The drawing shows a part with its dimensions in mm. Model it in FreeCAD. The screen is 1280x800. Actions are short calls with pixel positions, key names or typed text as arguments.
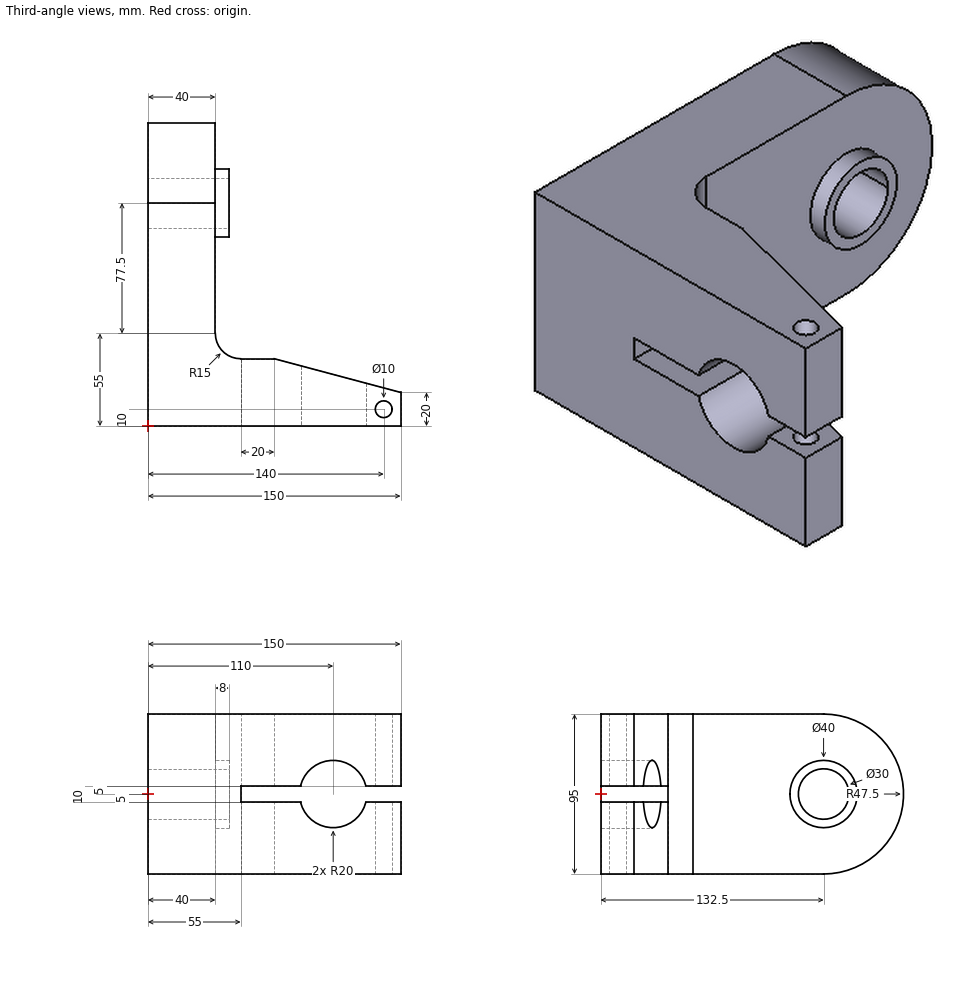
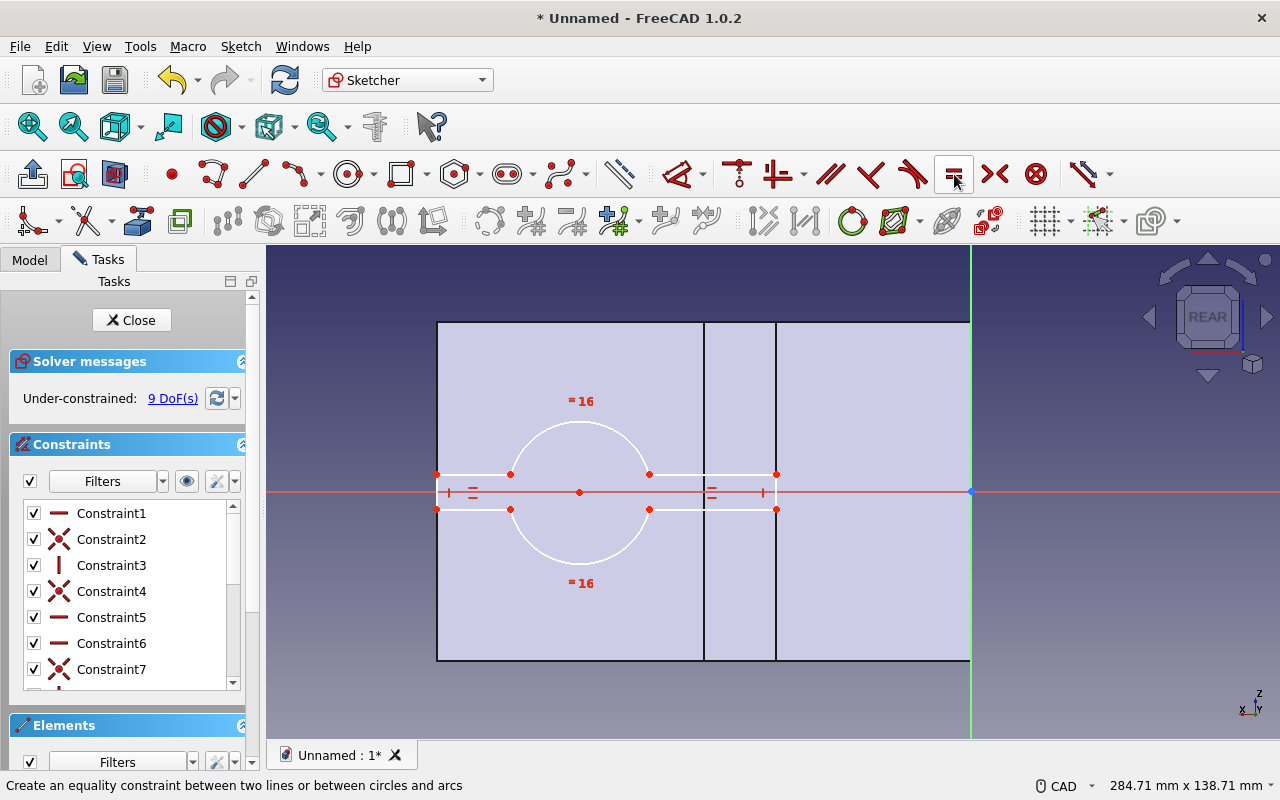
click(580, 493)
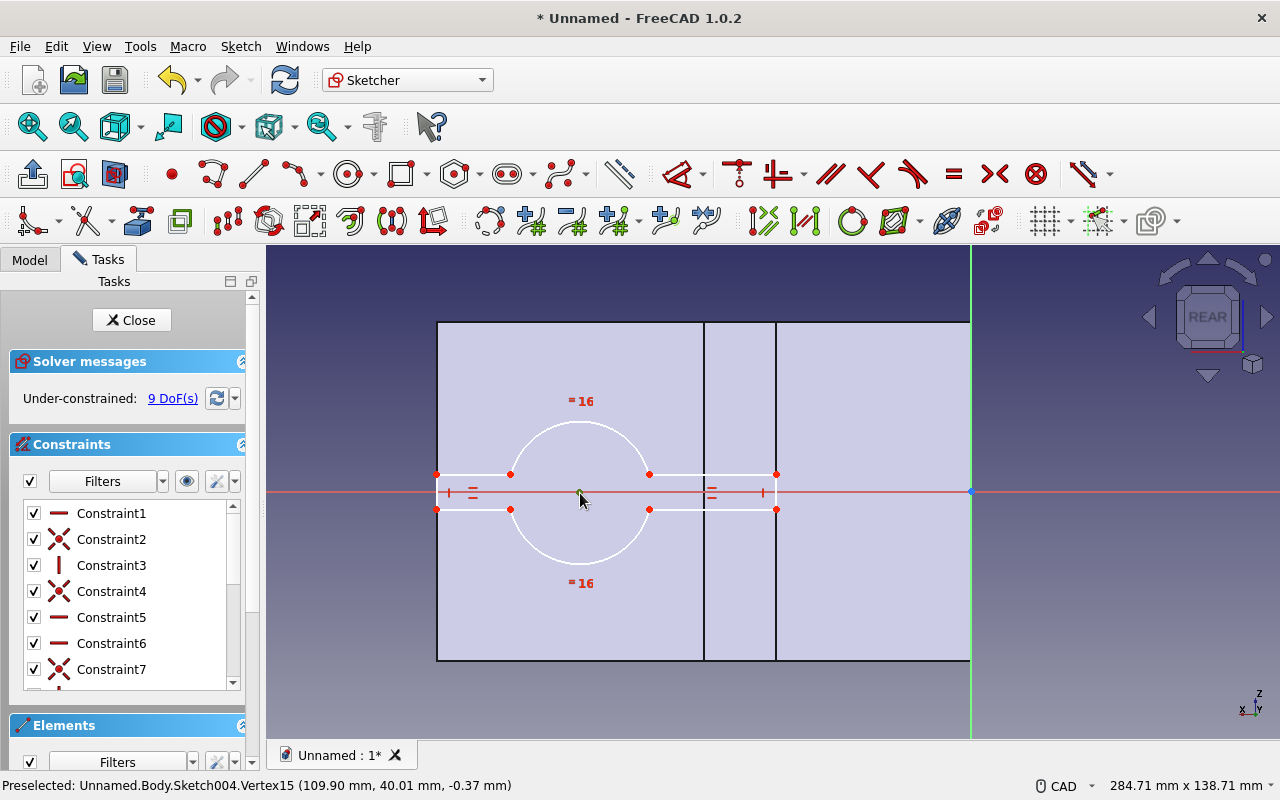
click(353, 492)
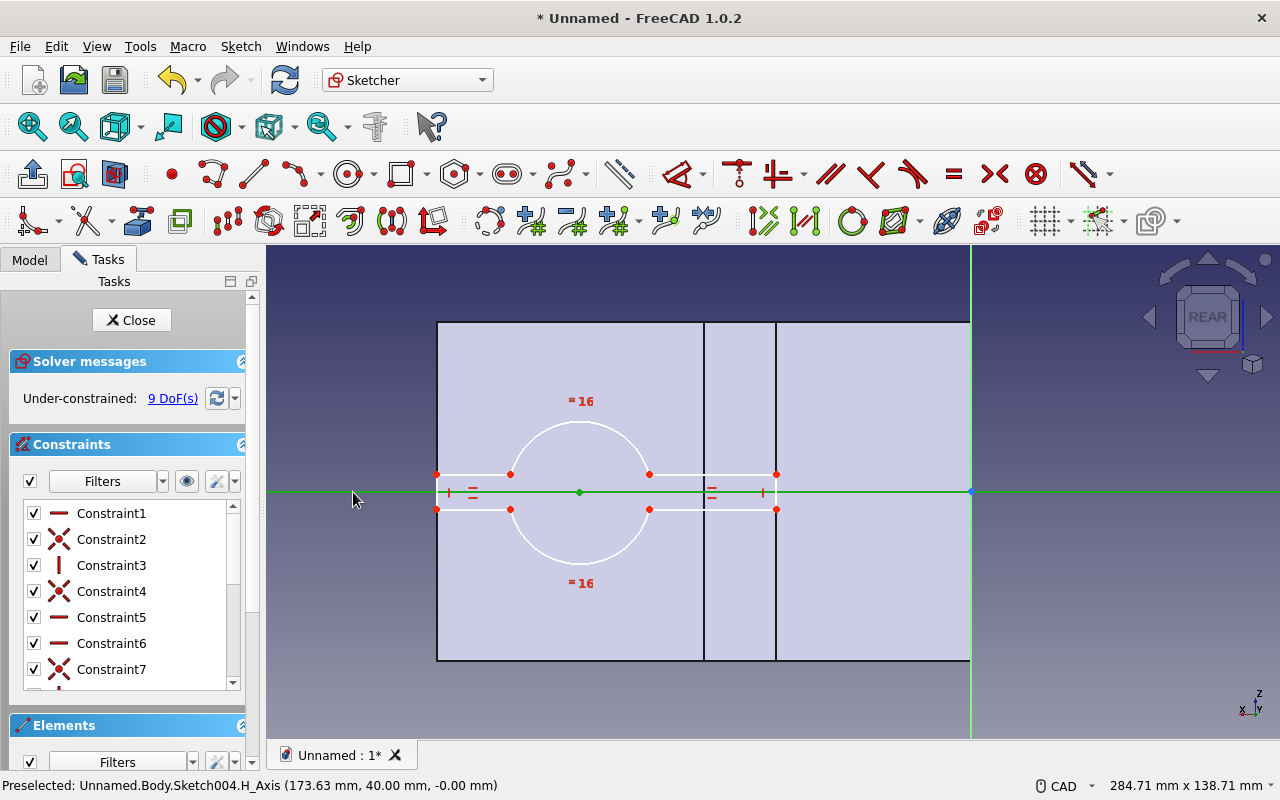
click(737, 174)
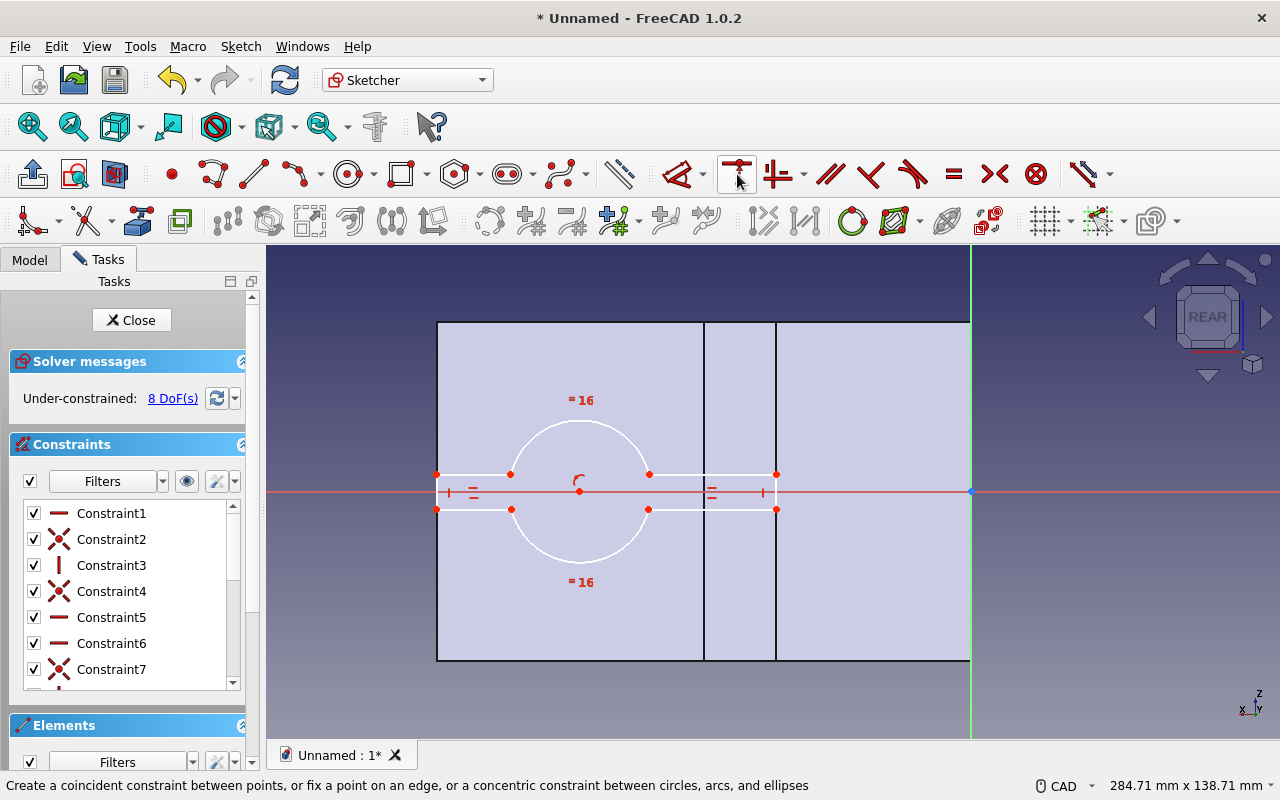
click(676, 174)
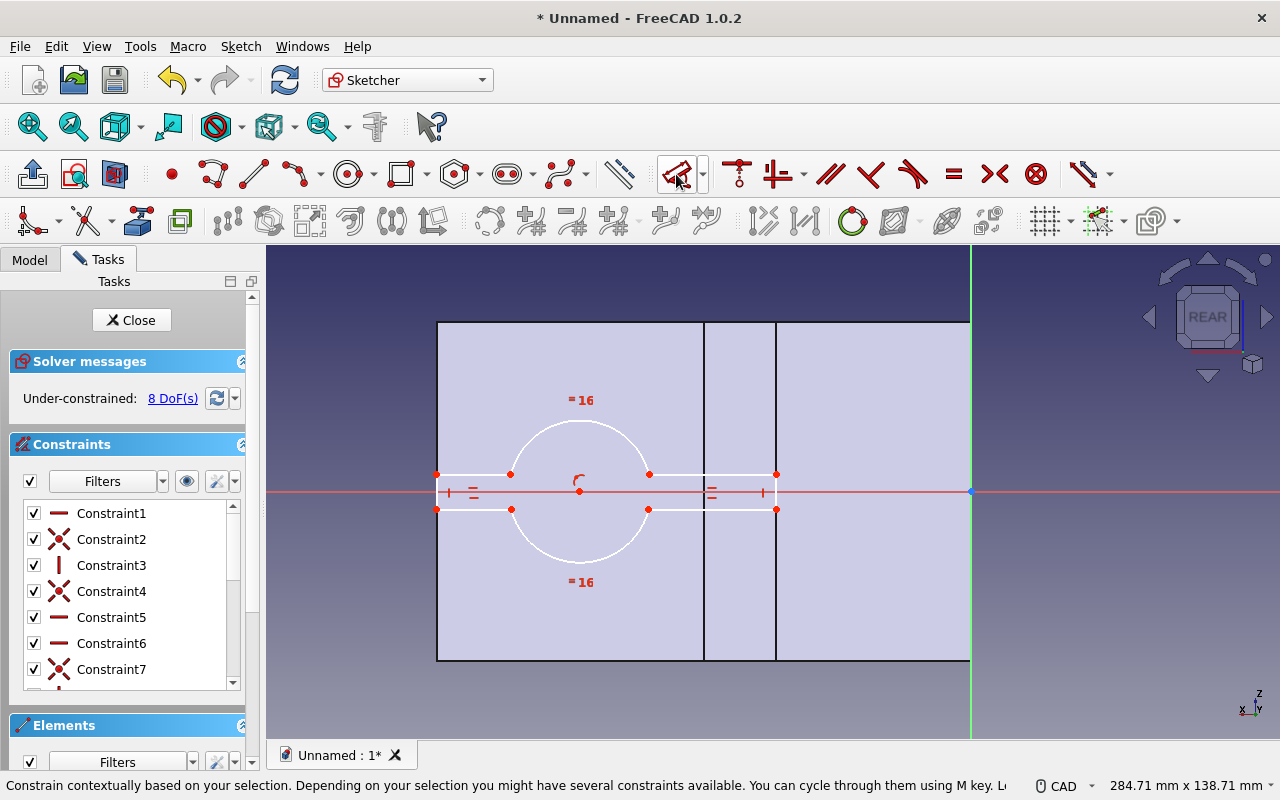
click(616, 430)
click(632, 402)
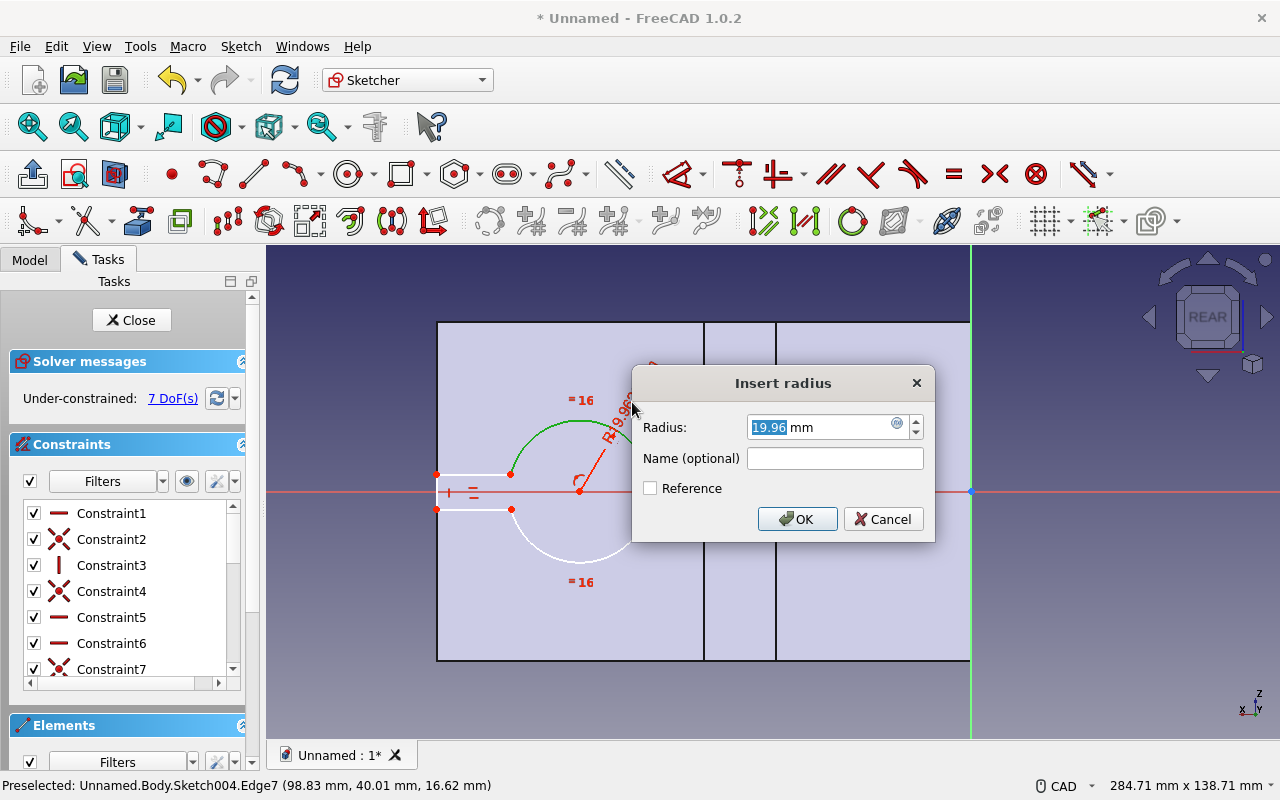
text(20)
key(Return)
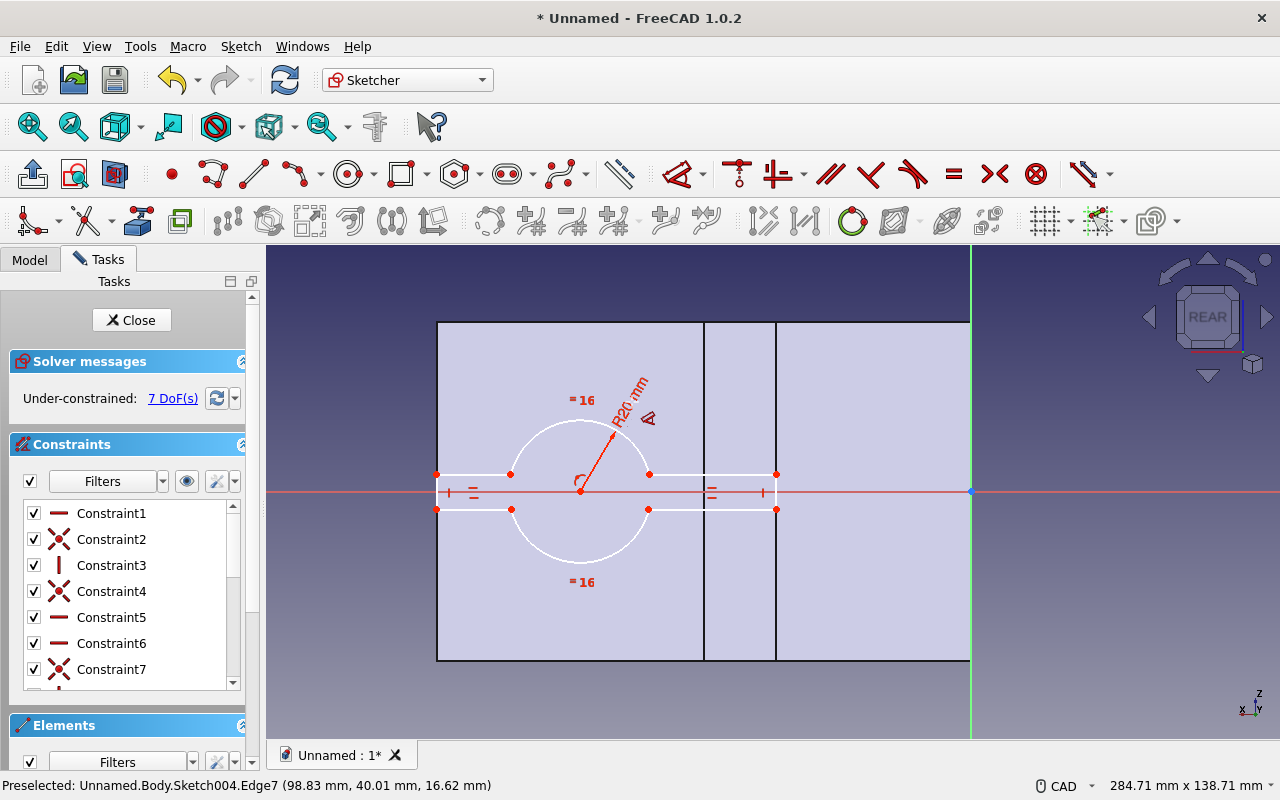
click(776, 489)
click(810, 505)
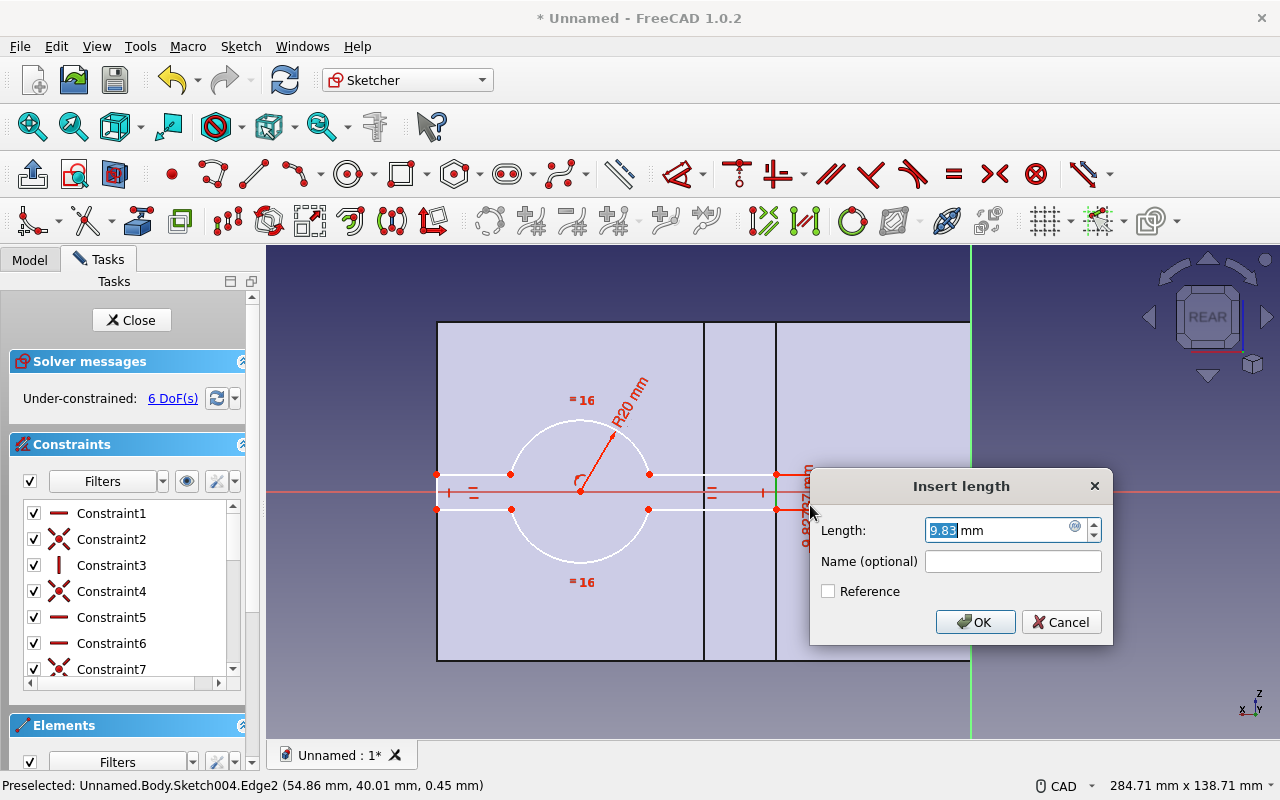
text(10)
key(Return)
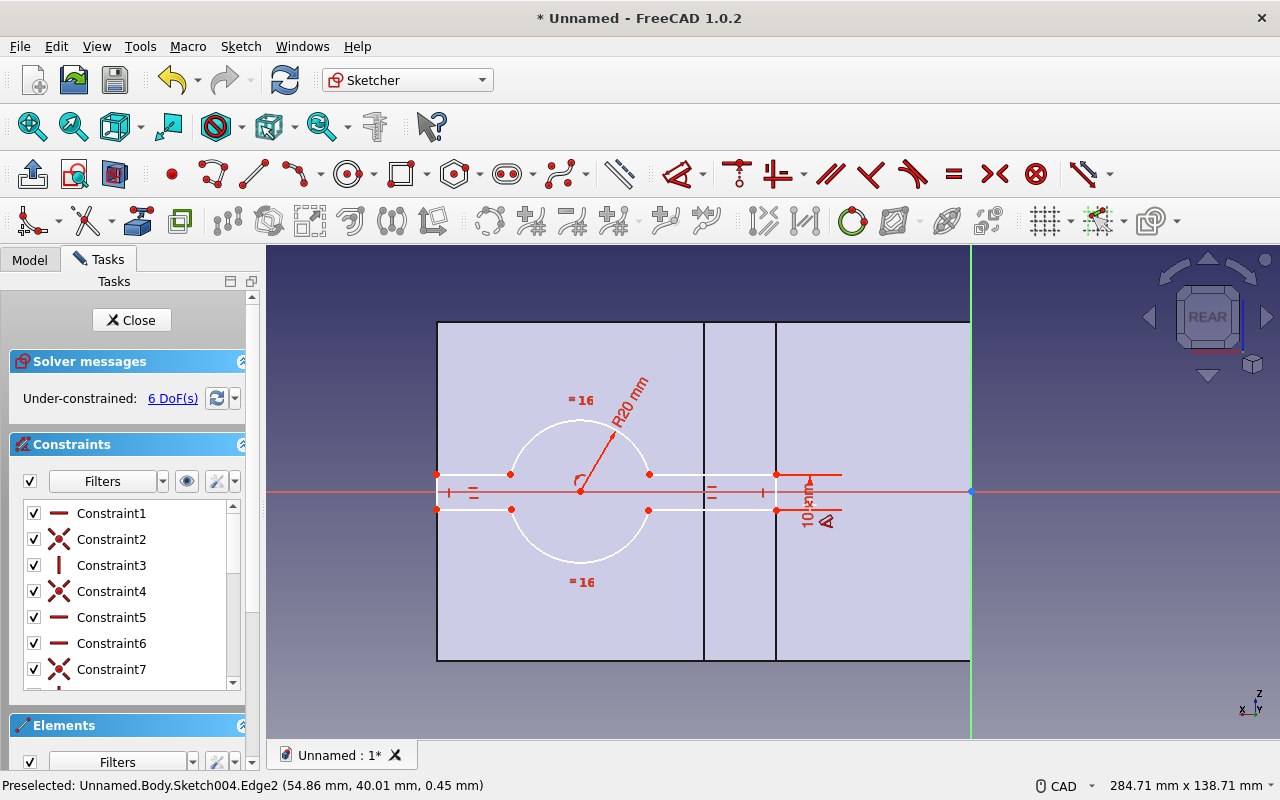
click(437, 489)
click(403, 505)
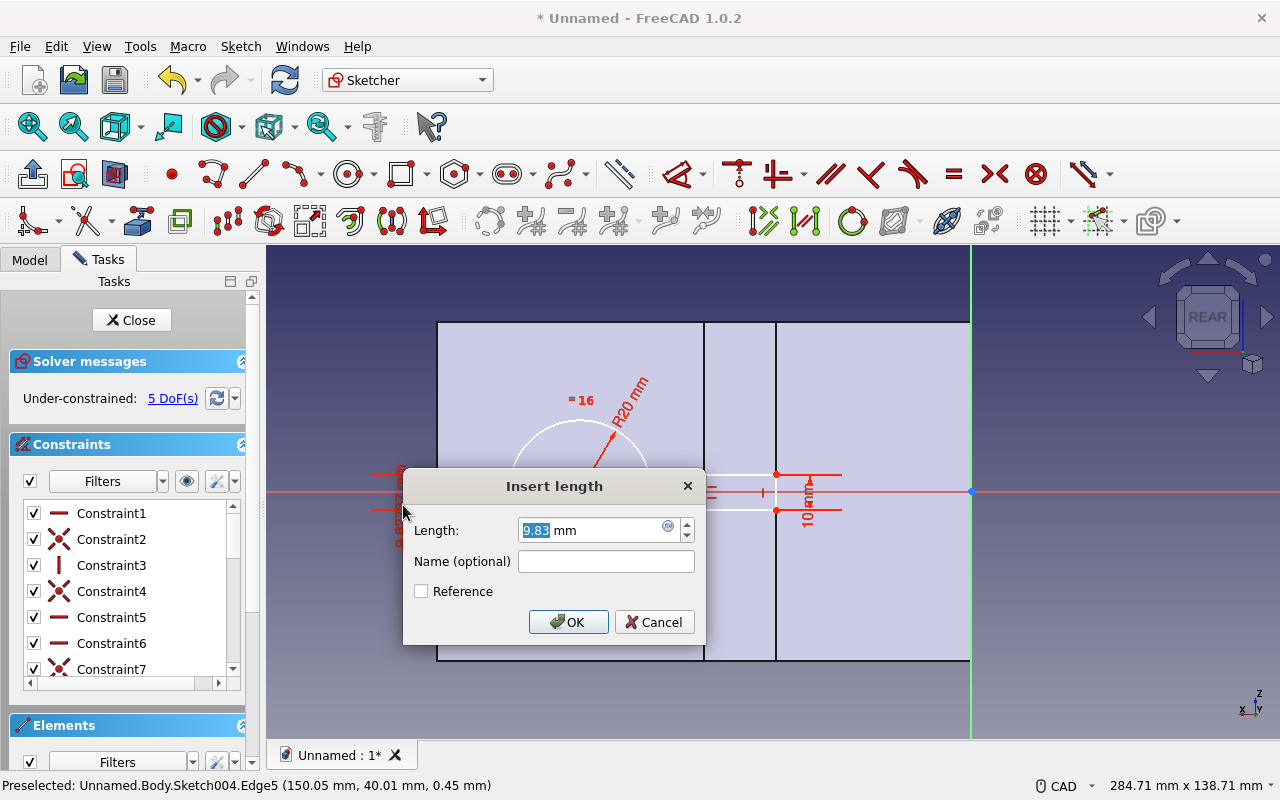
text(10)
key(Return)